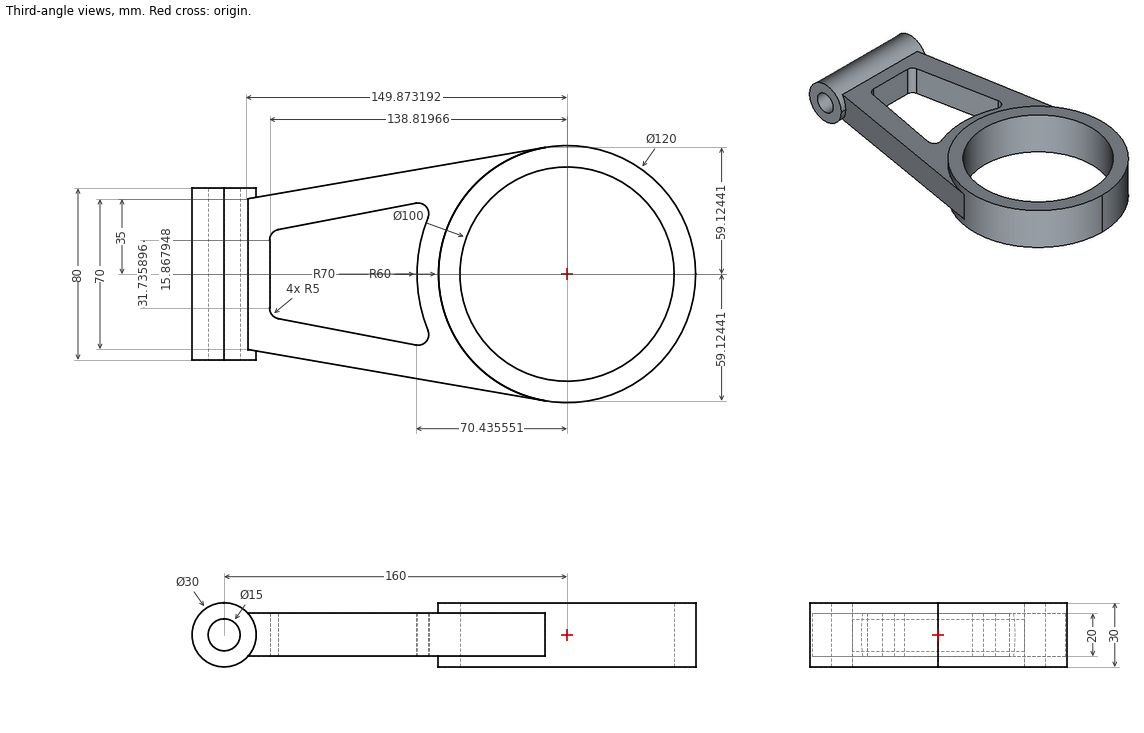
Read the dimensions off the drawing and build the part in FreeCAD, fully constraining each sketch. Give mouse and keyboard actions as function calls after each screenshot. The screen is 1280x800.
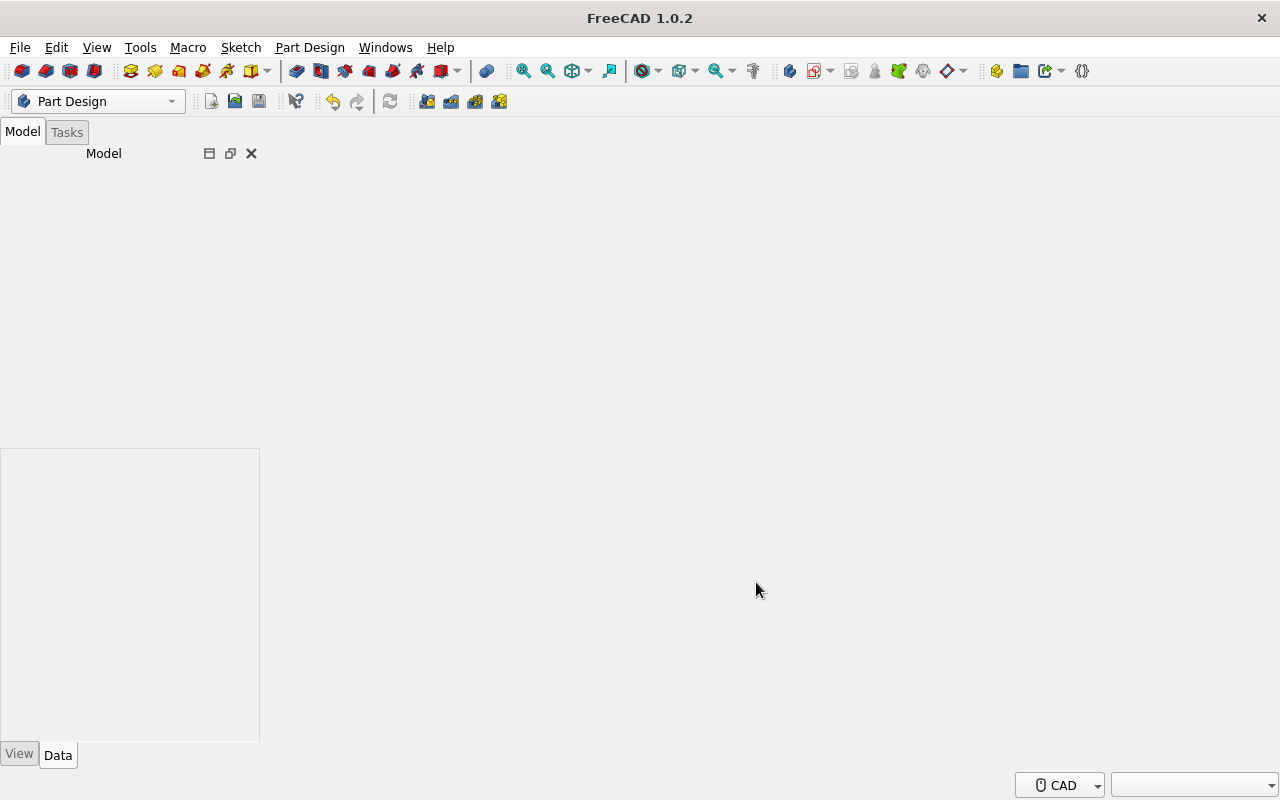
click(212, 102)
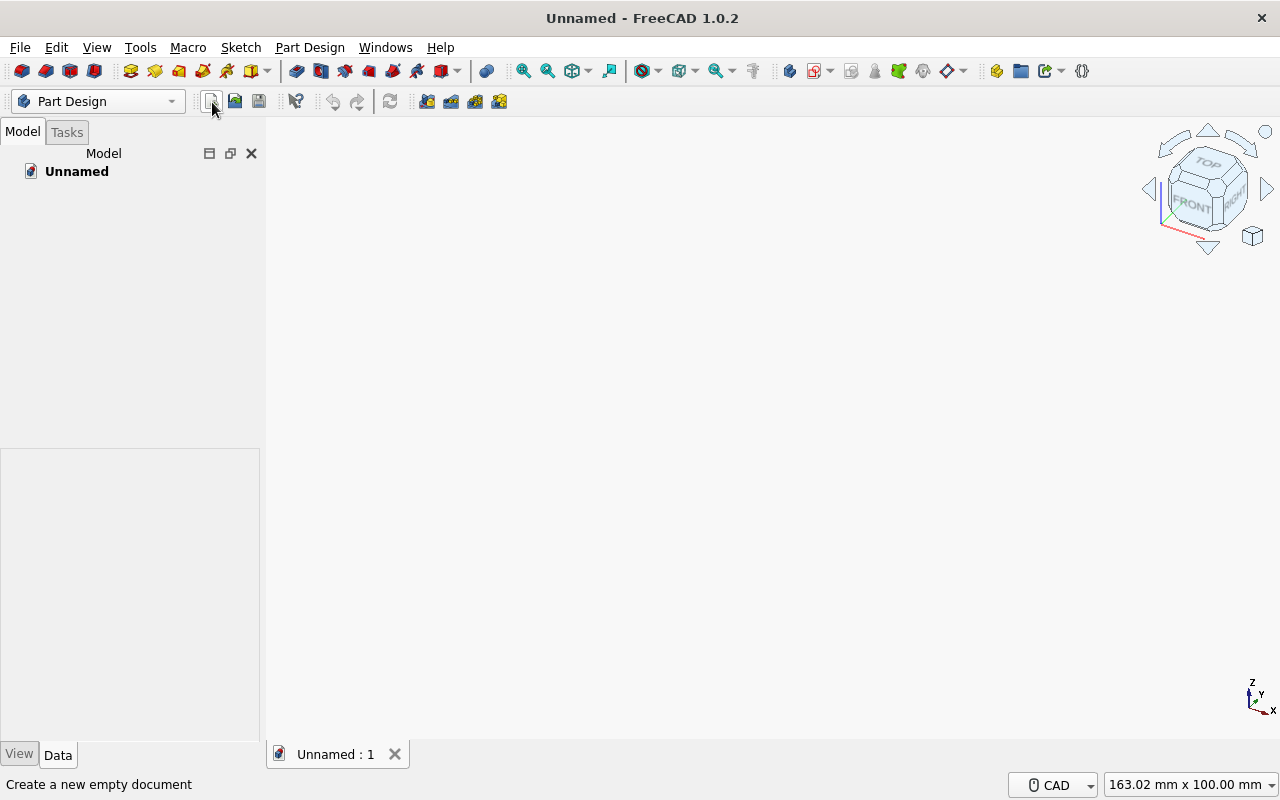
click(814, 72)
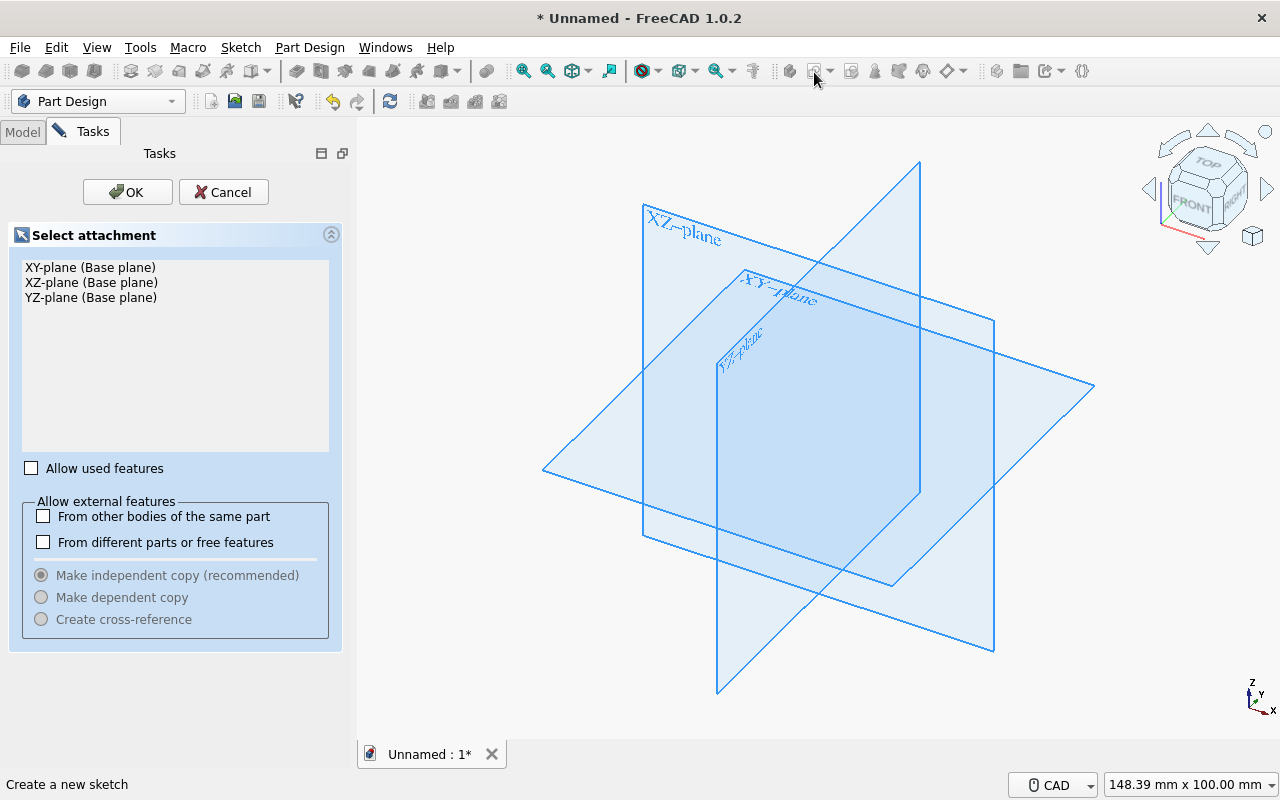
click(82, 268)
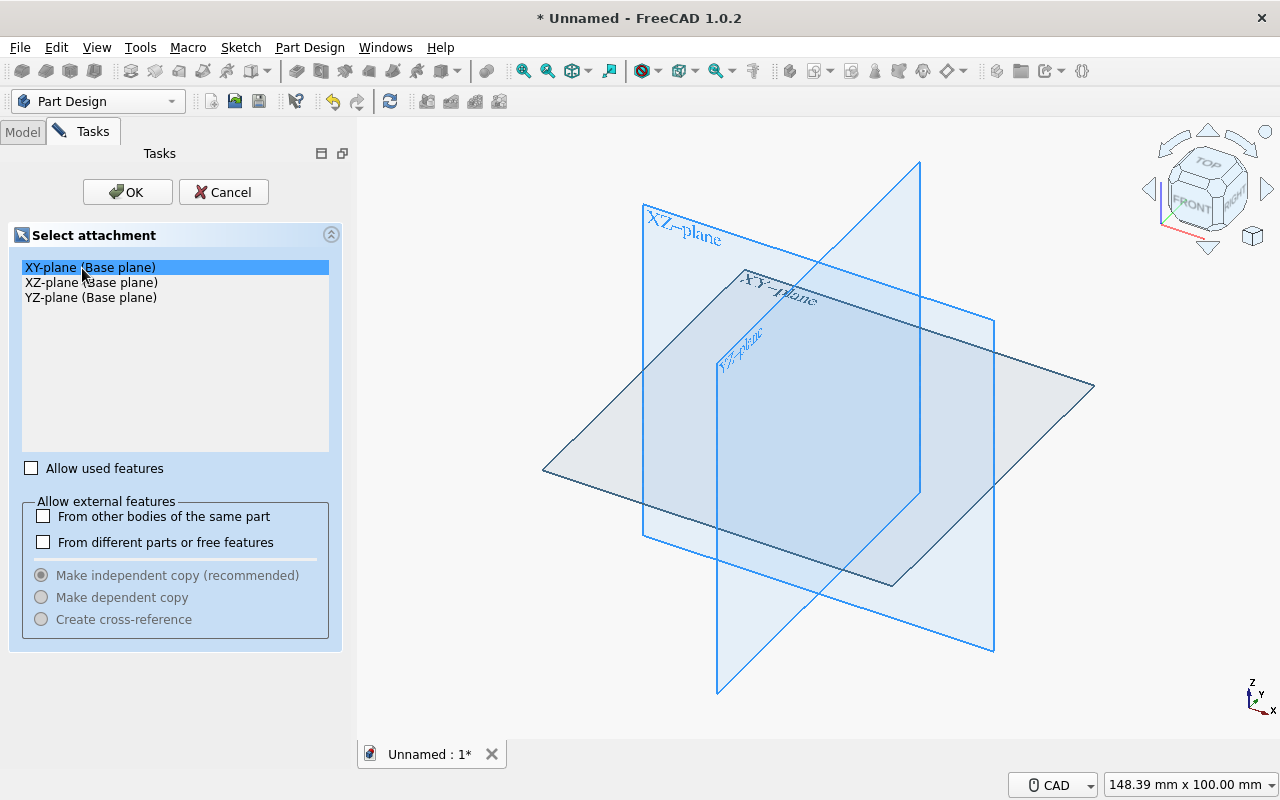
click(128, 192)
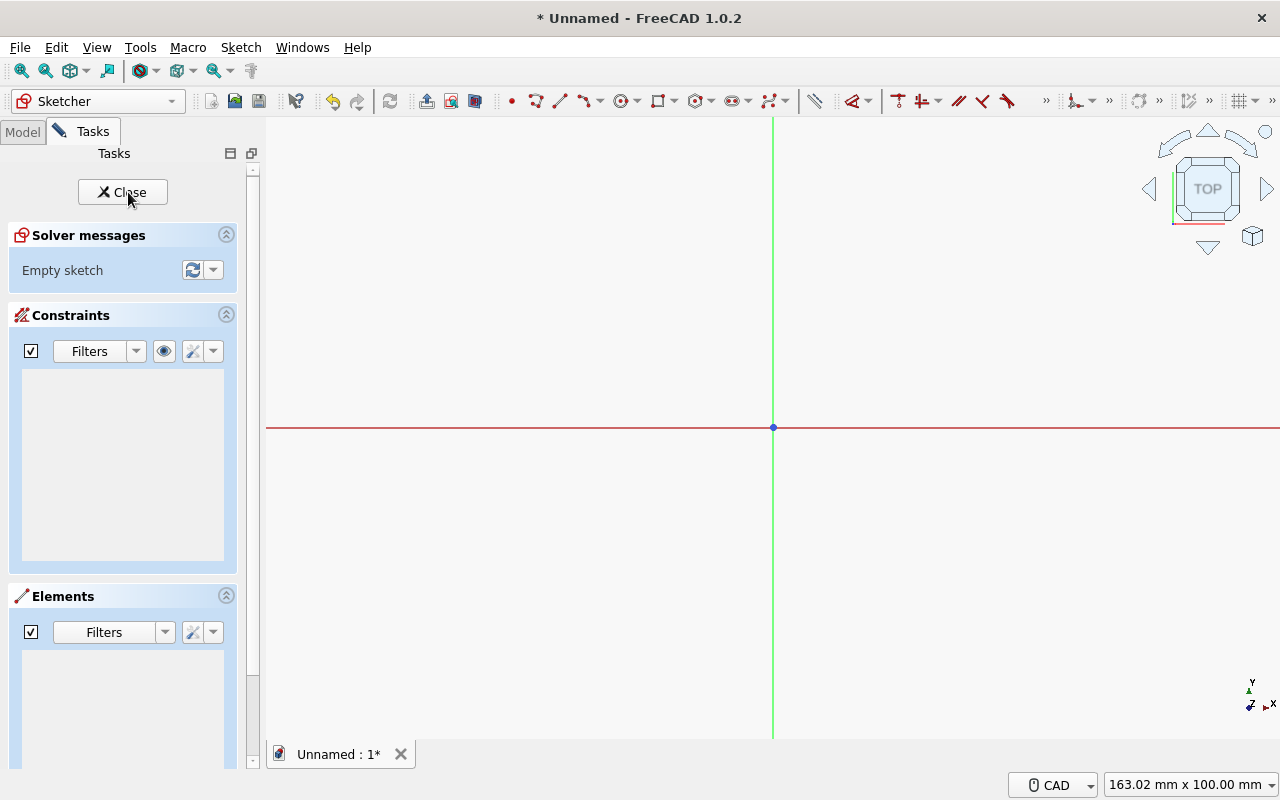
scroll(621, 428, down, 3)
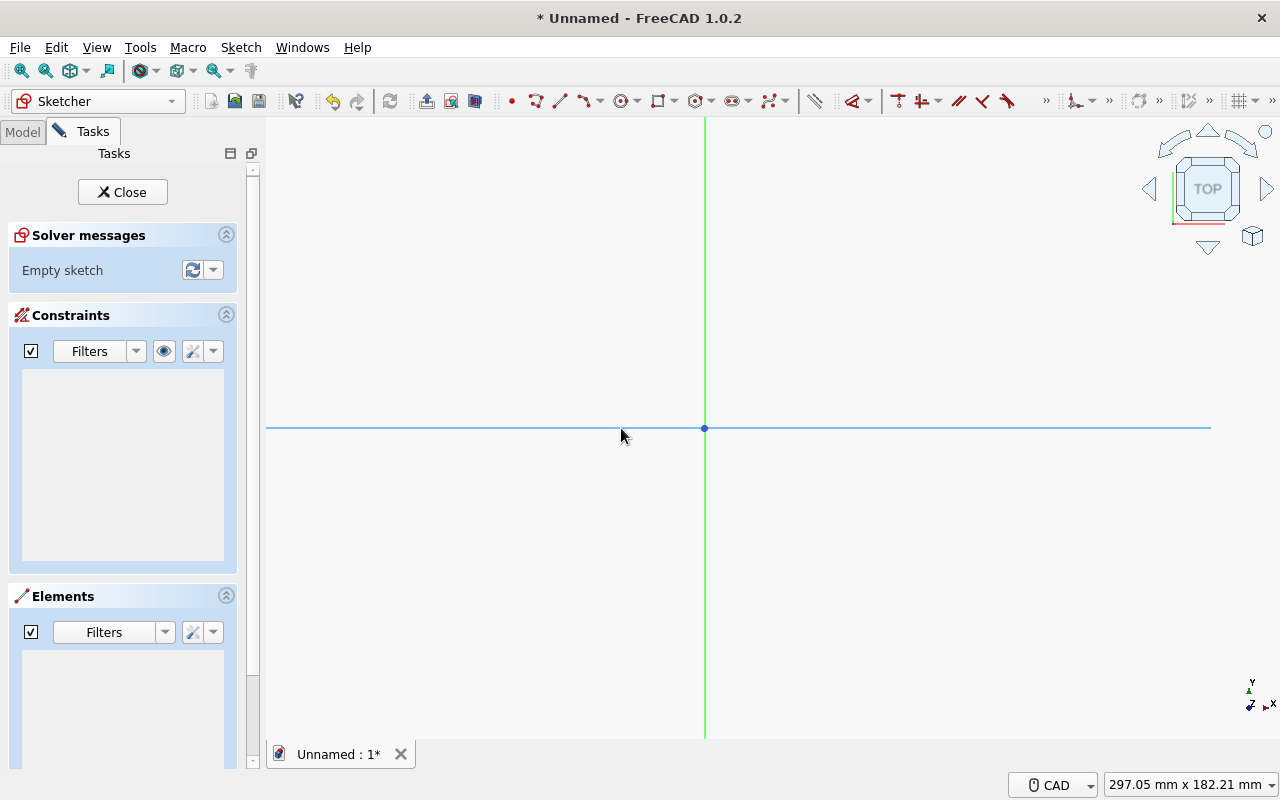
click(622, 102)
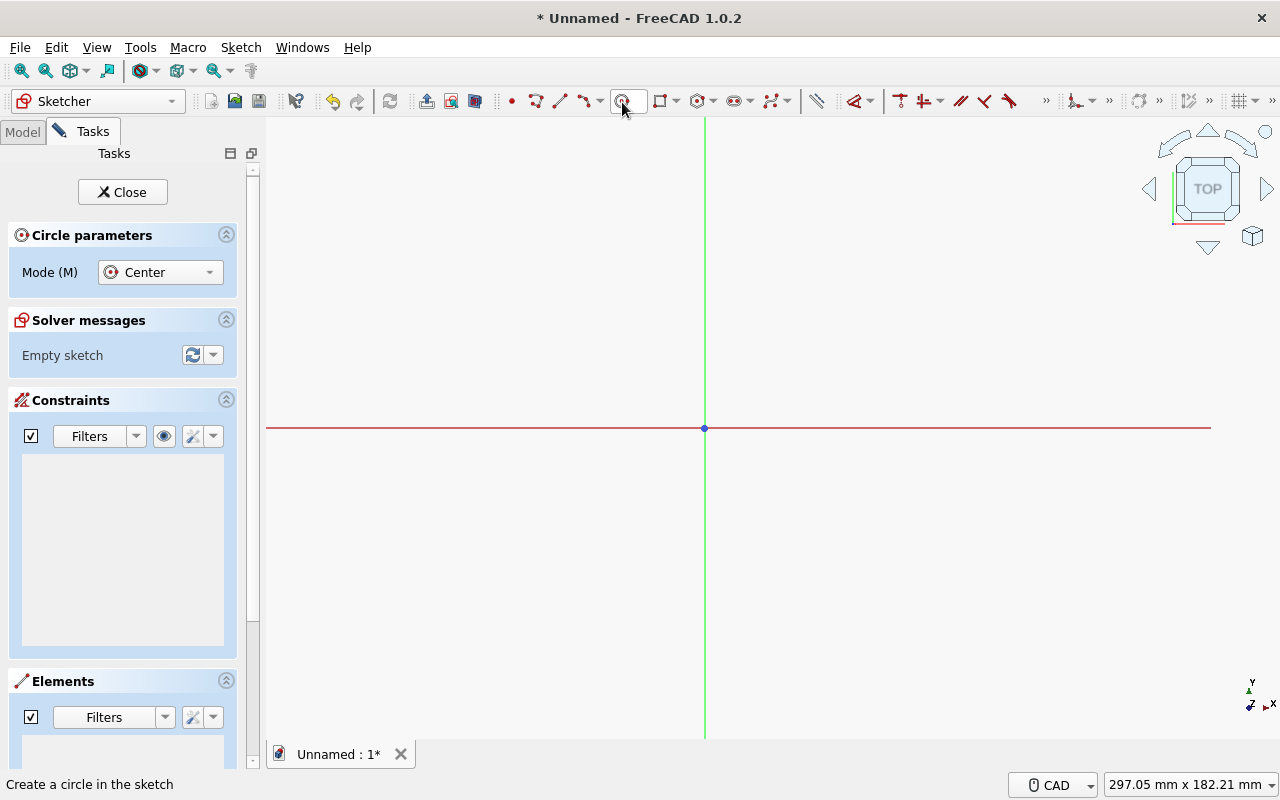
click(705, 428)
move(849, 283)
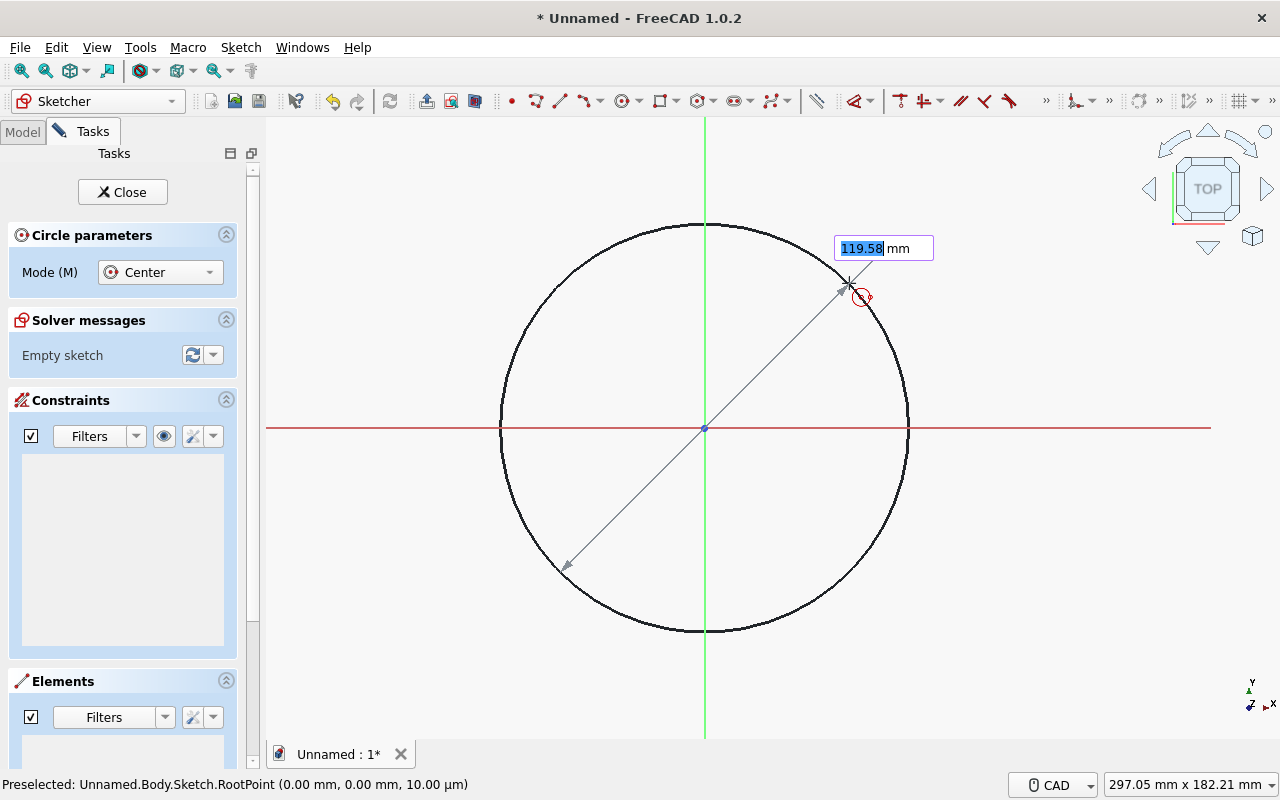
text(120)
key(Return)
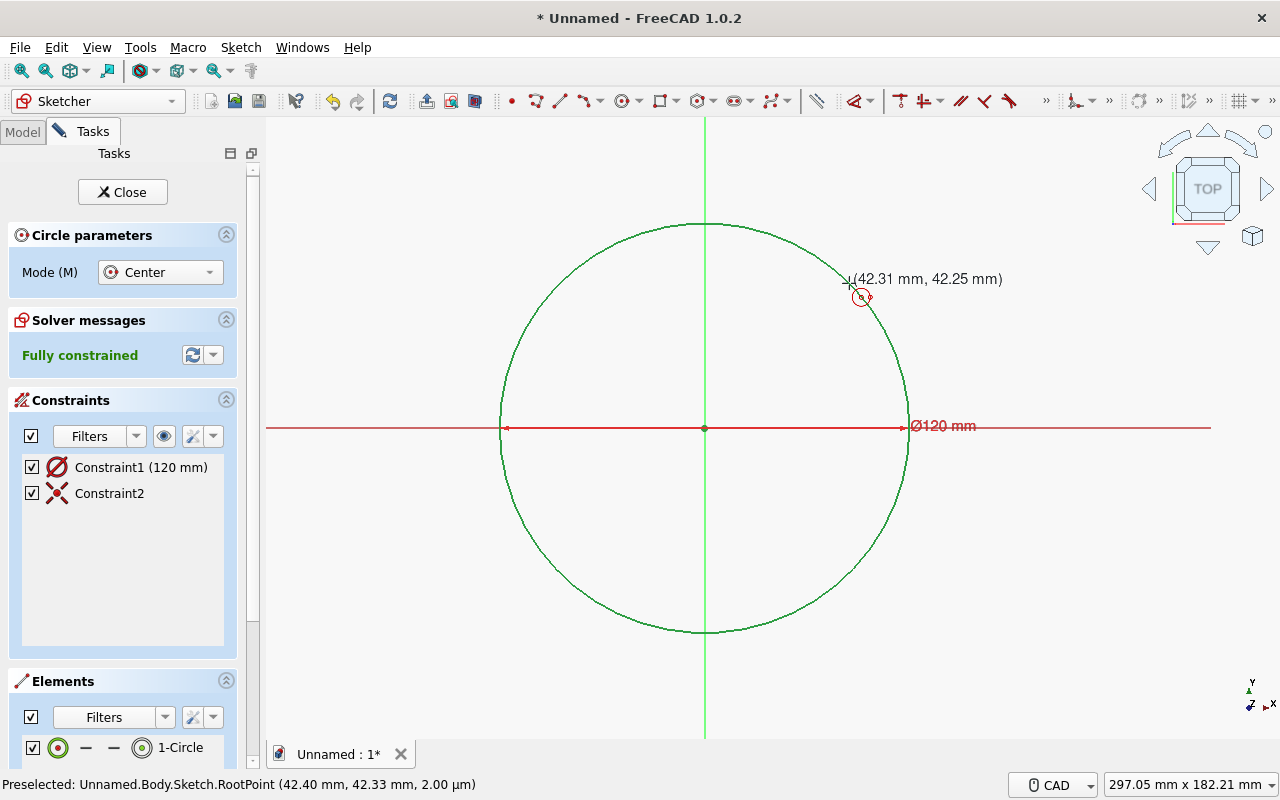
click(705, 428)
move(825, 308)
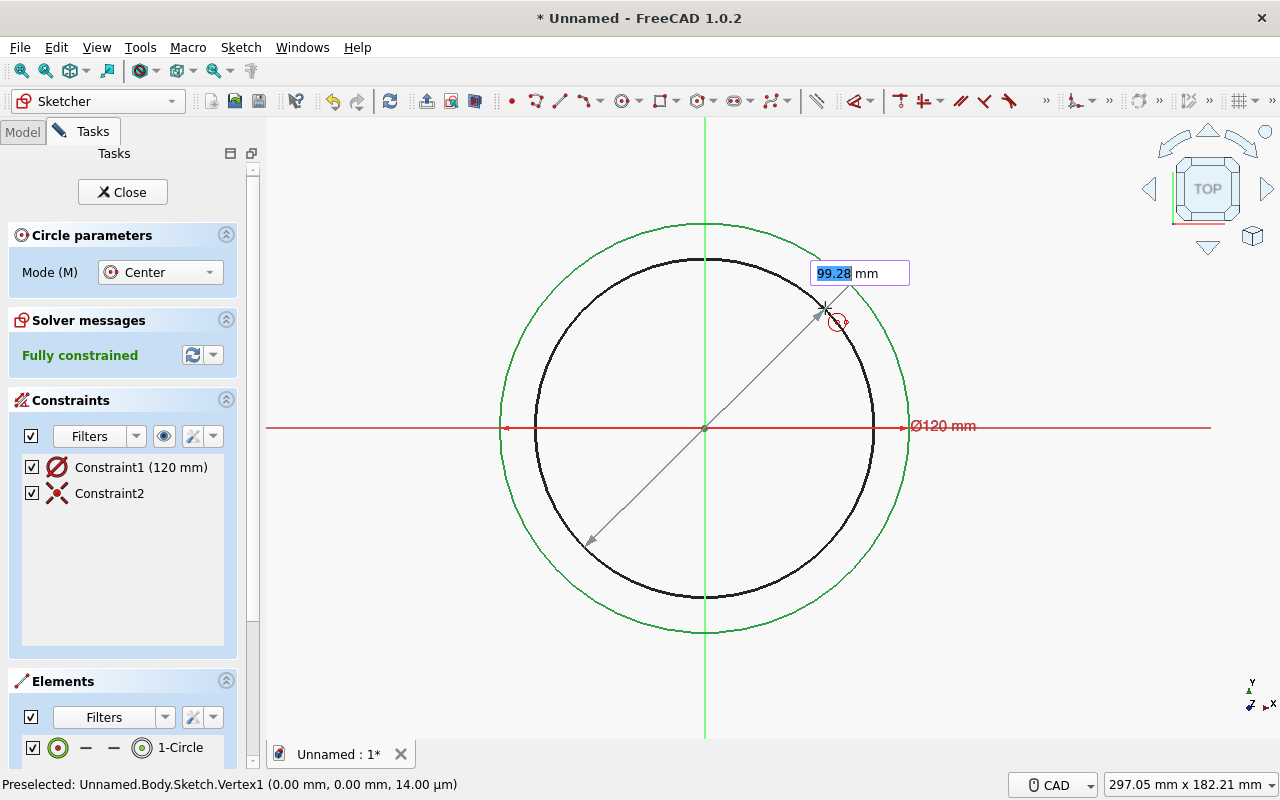
text(100)
key(Return)
key(Escape)